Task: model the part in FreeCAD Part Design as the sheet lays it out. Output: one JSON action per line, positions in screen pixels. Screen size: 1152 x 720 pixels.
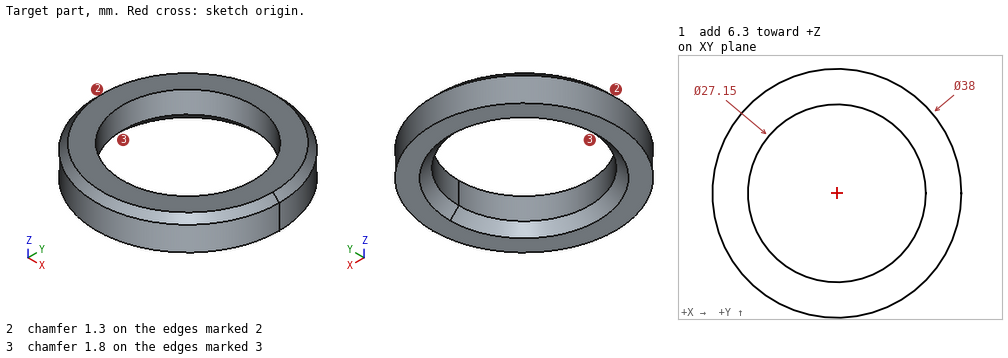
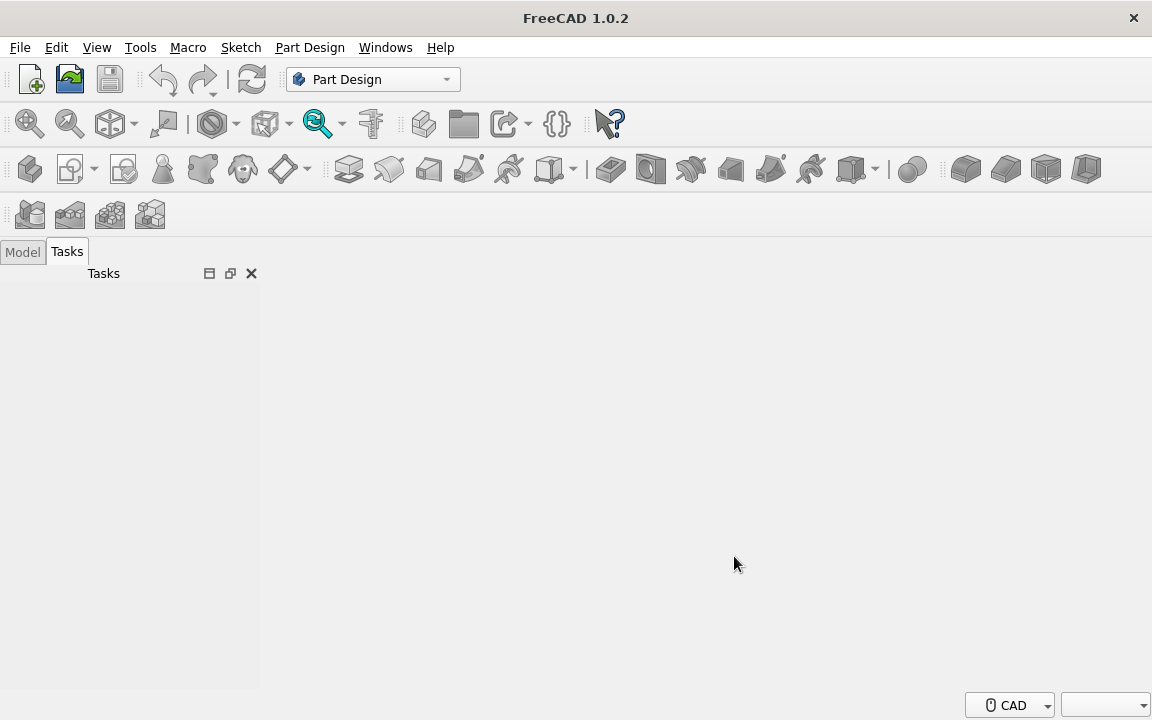
{"action": "left_click", "coordinate": [30, 80]}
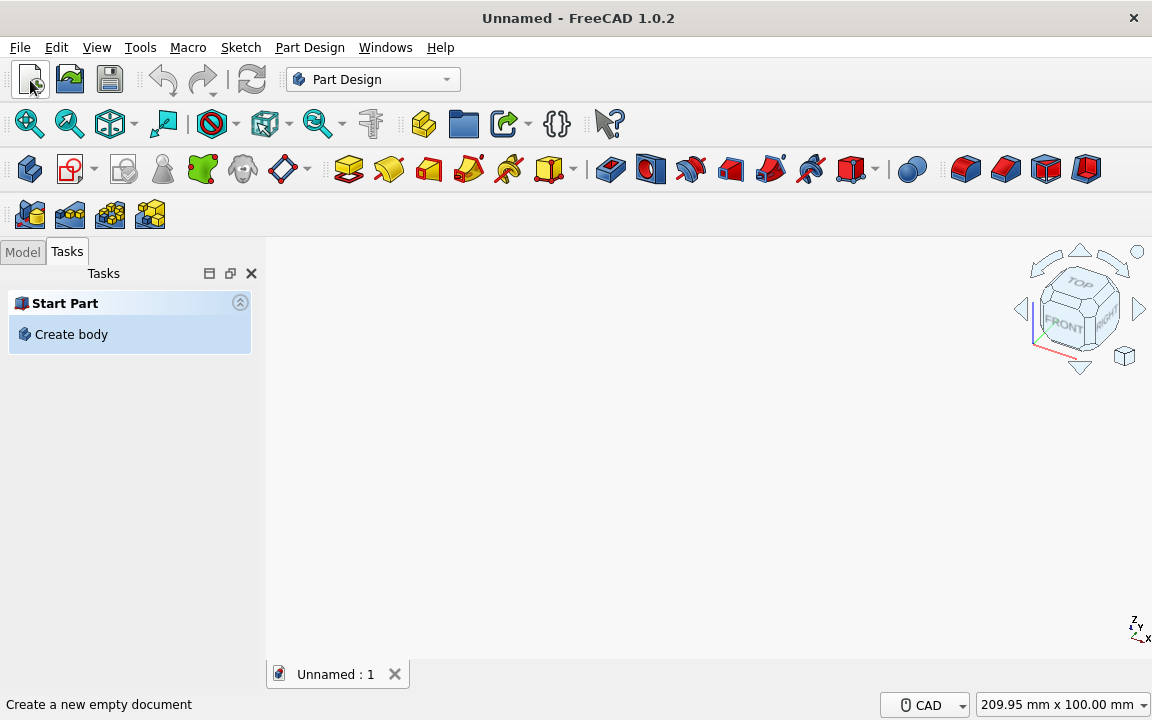
{"action": "left_click", "coordinate": [70, 170]}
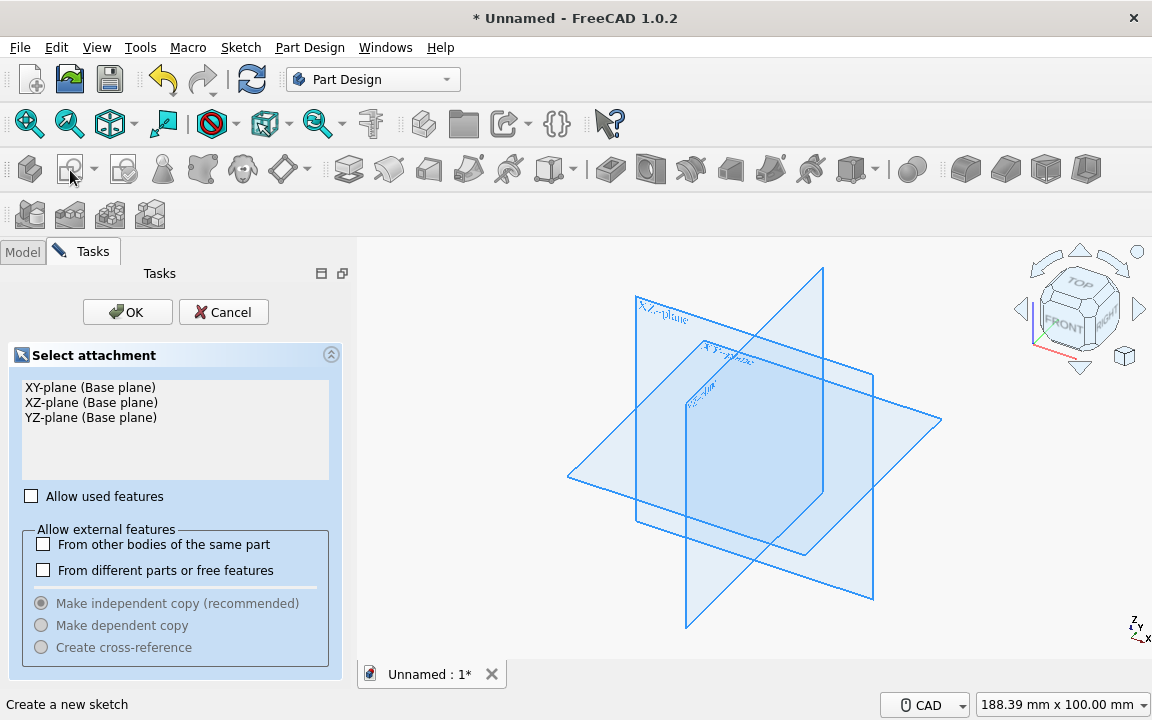
{"action": "left_click", "coordinate": [82, 388]}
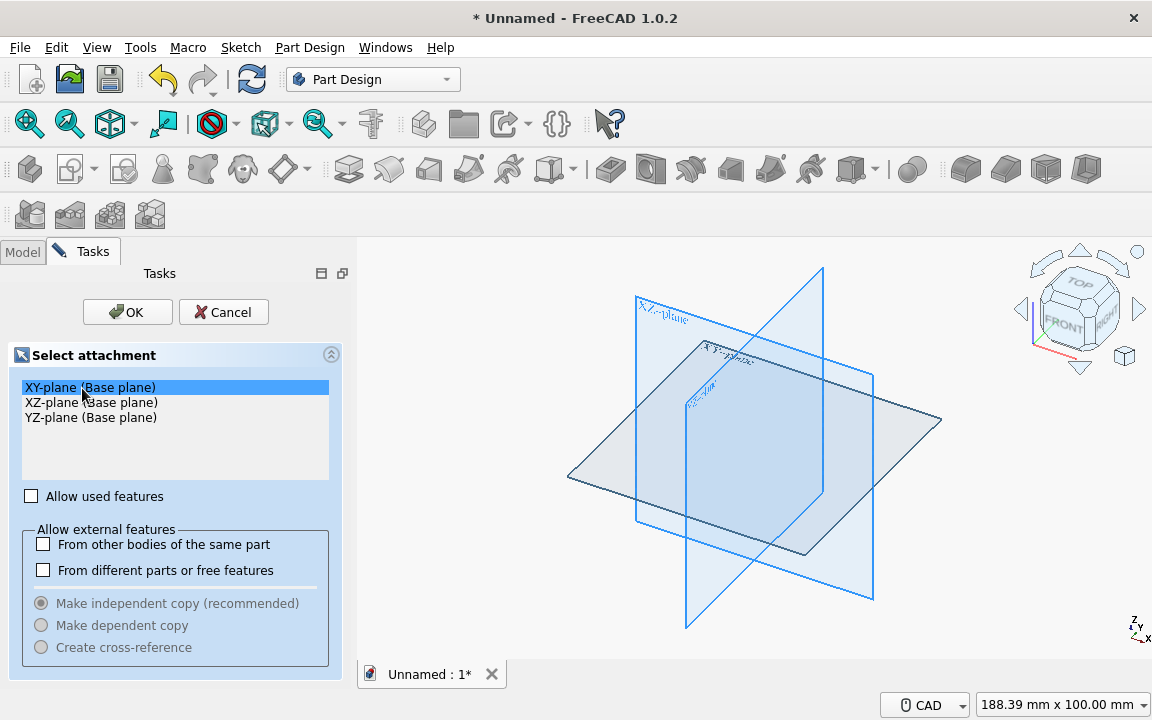
{"action": "left_click", "coordinate": [128, 312]}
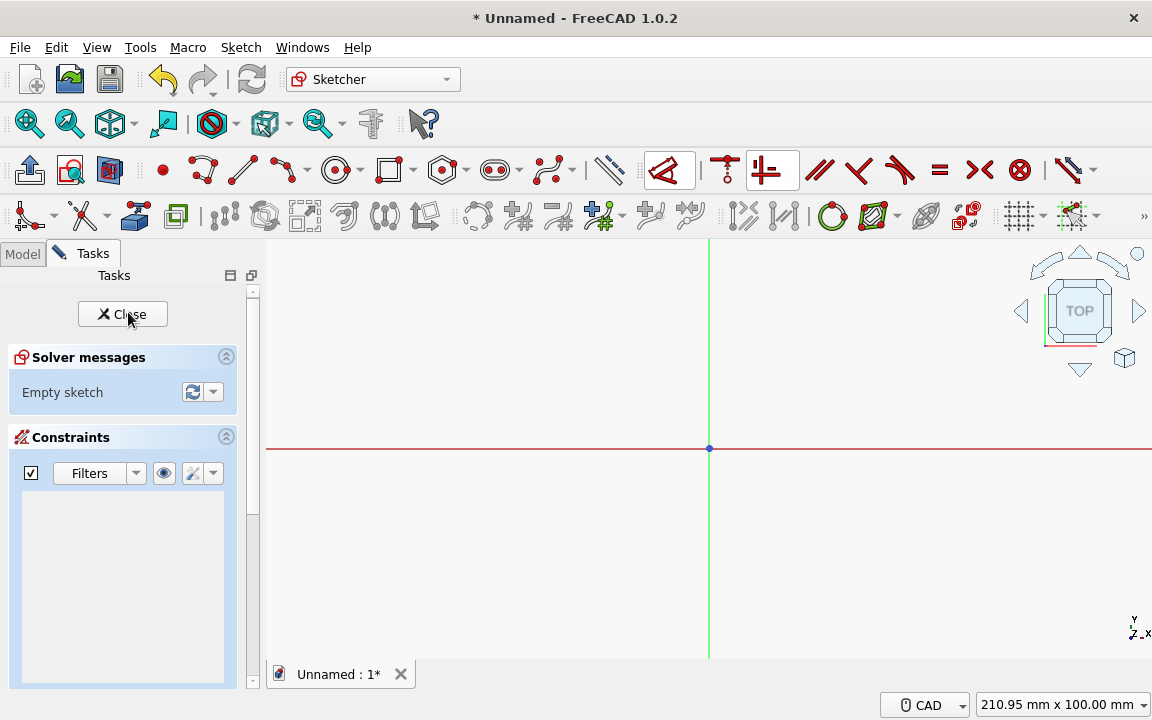
{"action": "scroll", "coordinate": [848, 449], "scroll_direction": "up", "scroll_amount": 2}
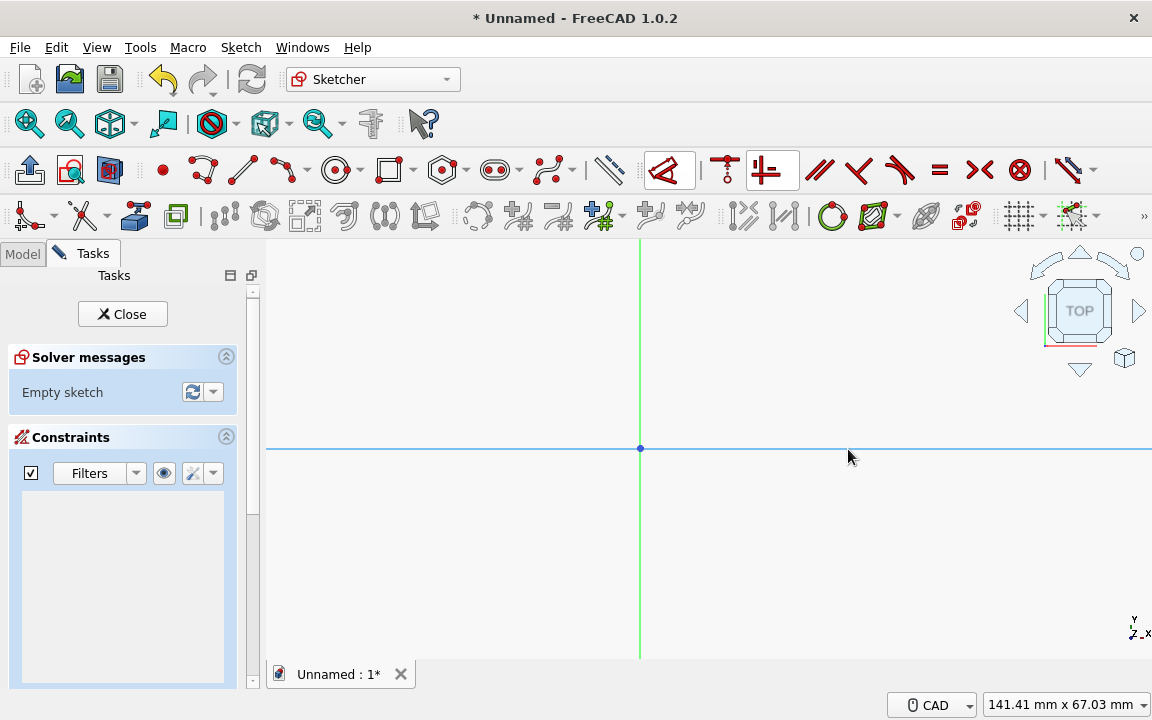
{"action": "key", "text": "g c"}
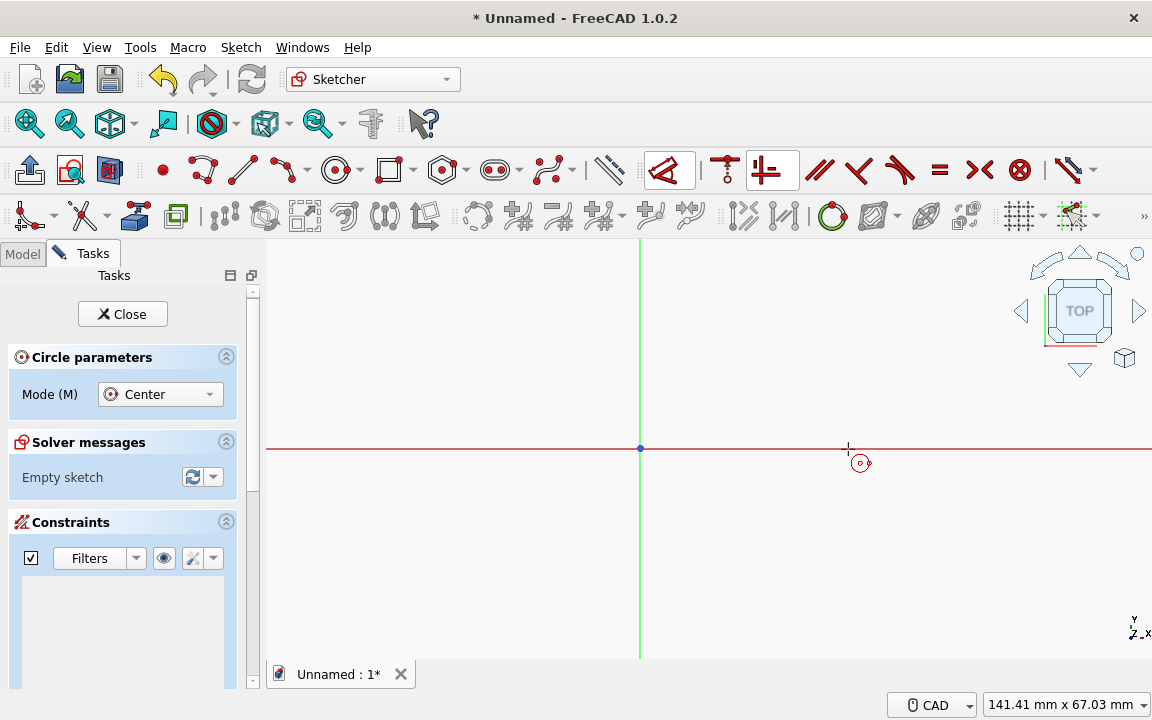
{"action": "left_click", "coordinate": [640, 449]}
{"action": "mouse_move", "coordinate": [724, 365]}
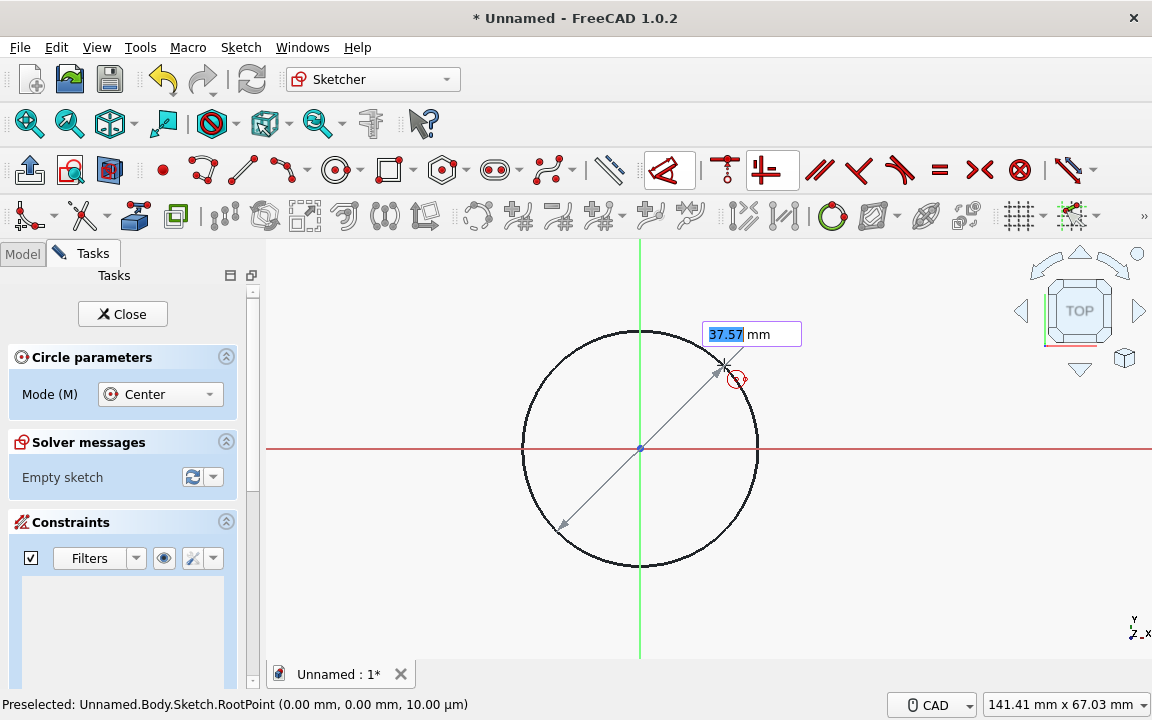
{"action": "type", "text": "38"}
{"action": "key", "text": "Return"}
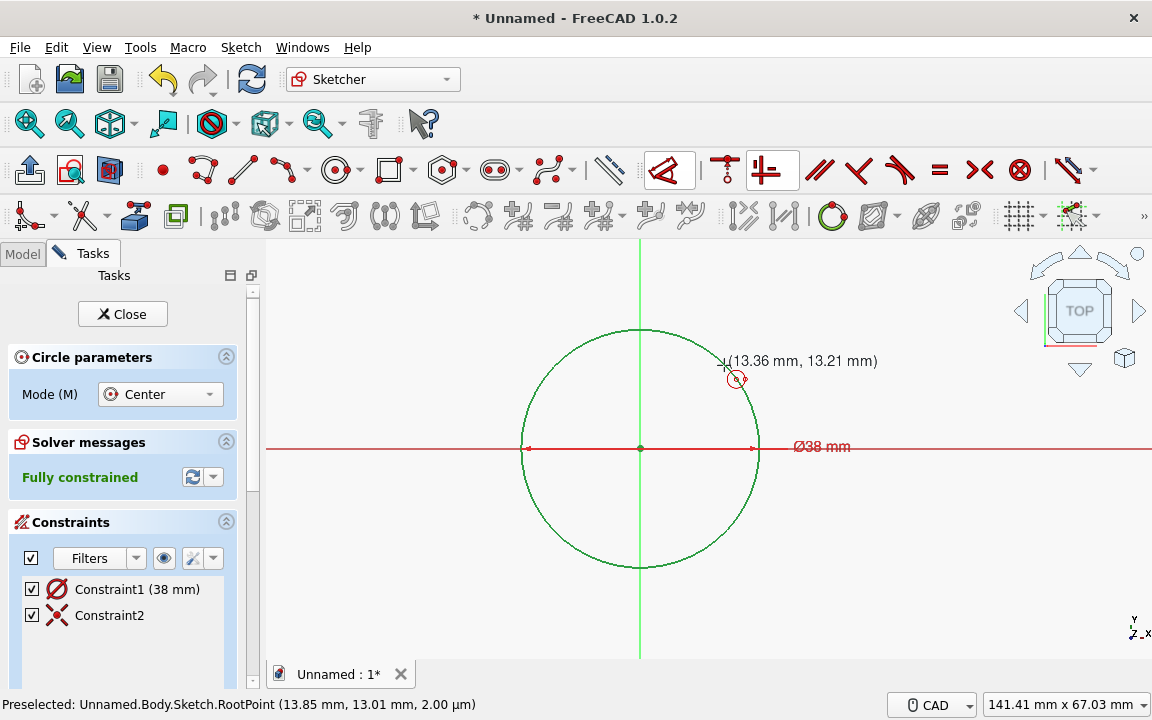
{"action": "left_click", "coordinate": [640, 449]}
{"action": "mouse_move", "coordinate": [700, 389]}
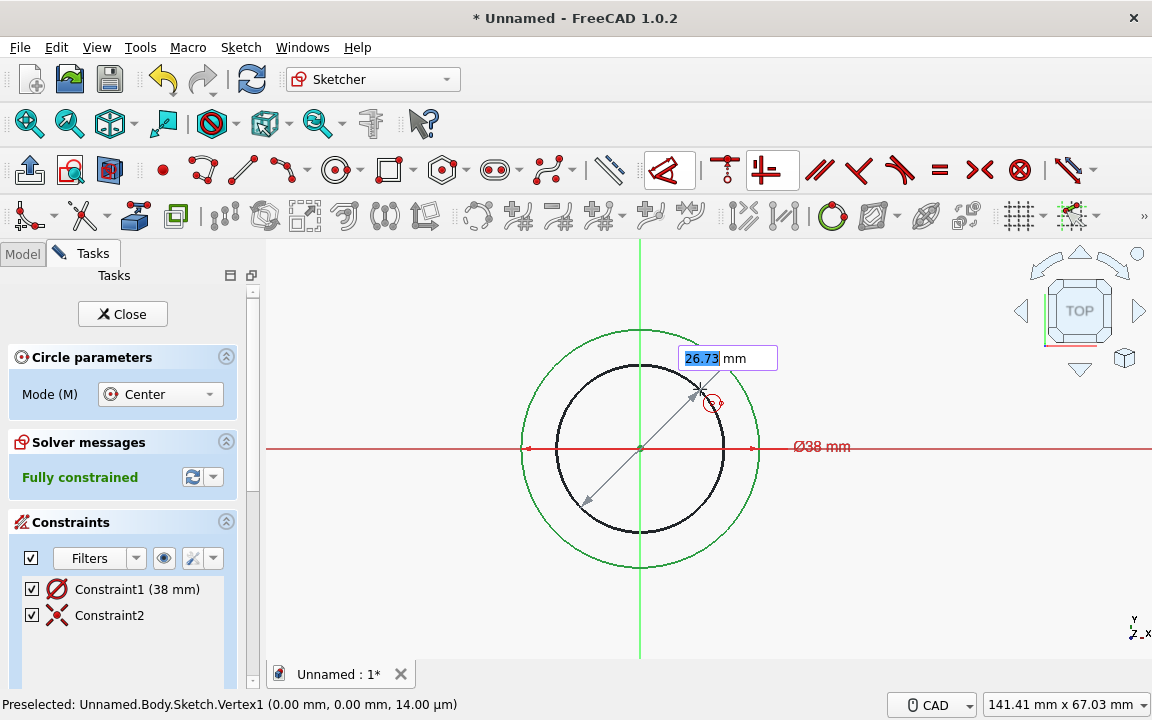
{"action": "type", "text": "27.15"}
{"action": "key", "text": "Return"}
{"action": "key", "text": "Escape"}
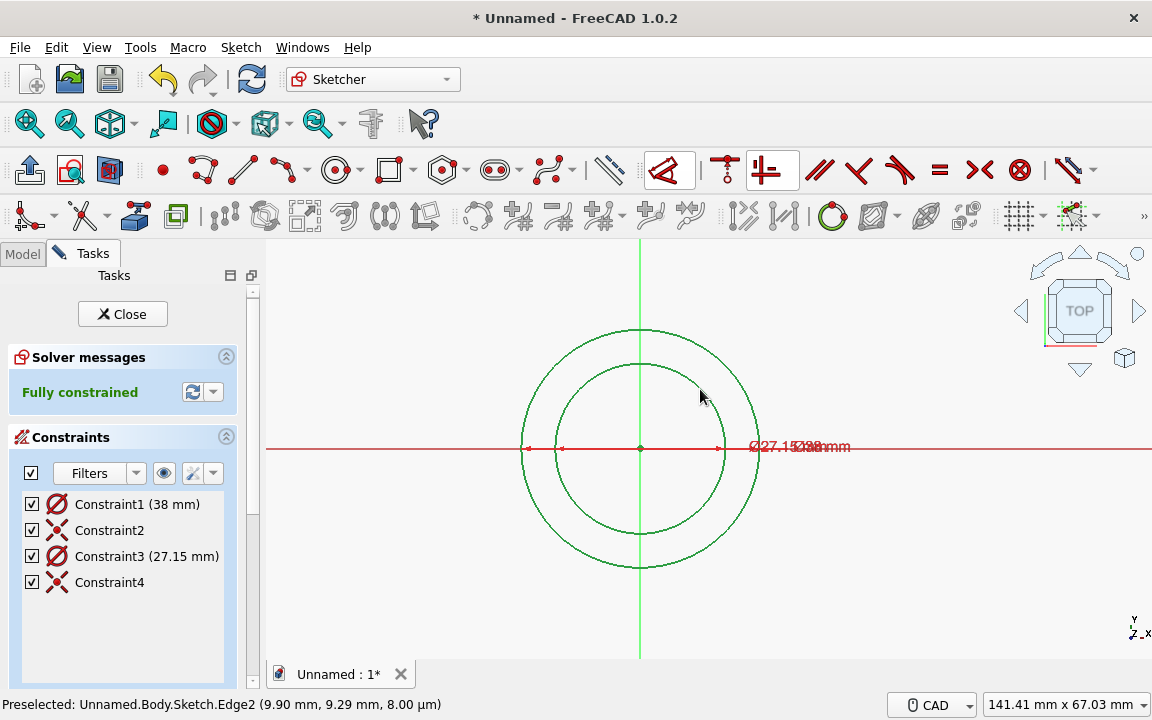
{"action": "left_click", "coordinate": [123, 314]}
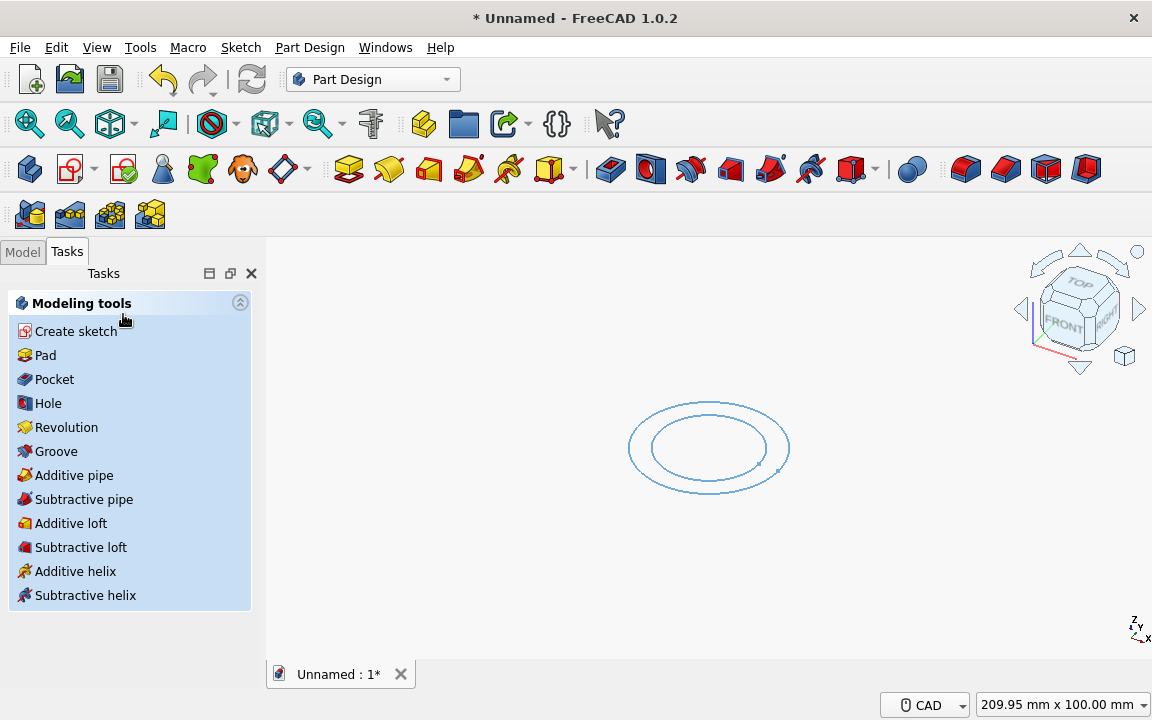
{"action": "left_click", "coordinate": [350, 170]}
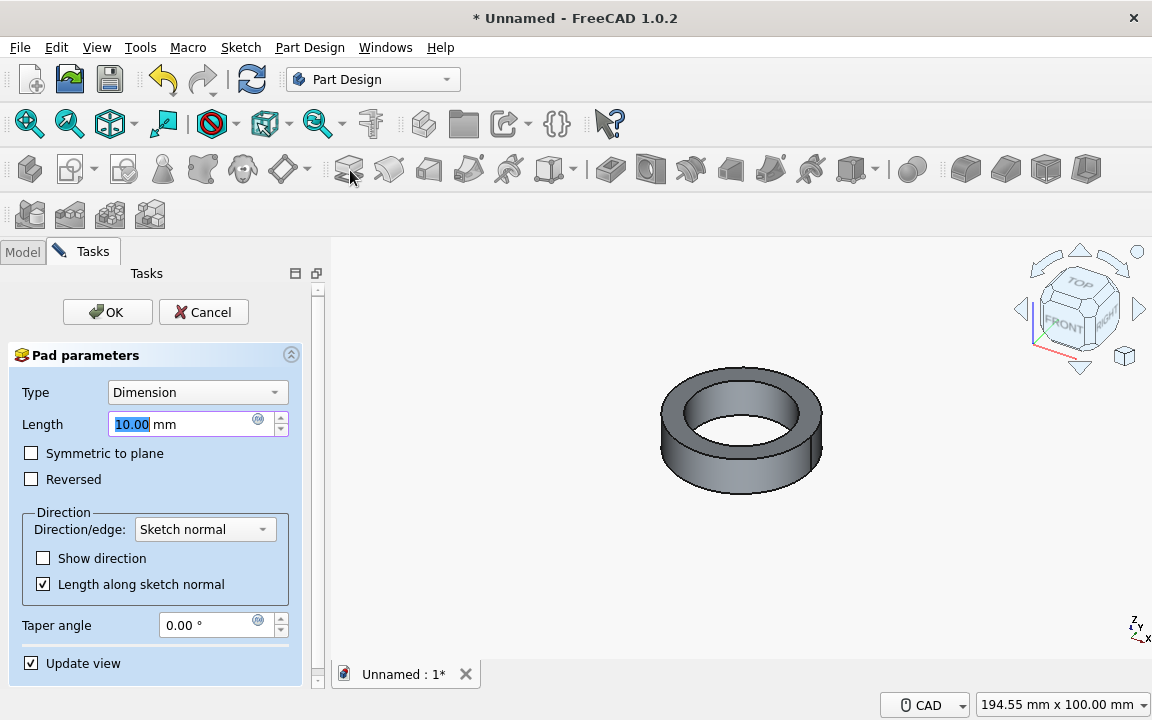
{"action": "type", "text": "6.3"}
{"action": "key", "text": "Tab"}